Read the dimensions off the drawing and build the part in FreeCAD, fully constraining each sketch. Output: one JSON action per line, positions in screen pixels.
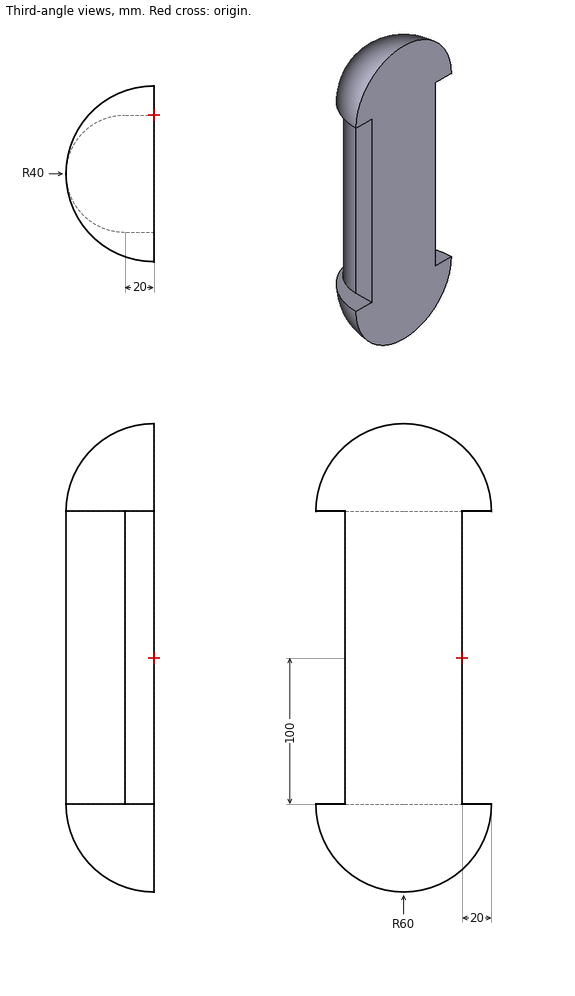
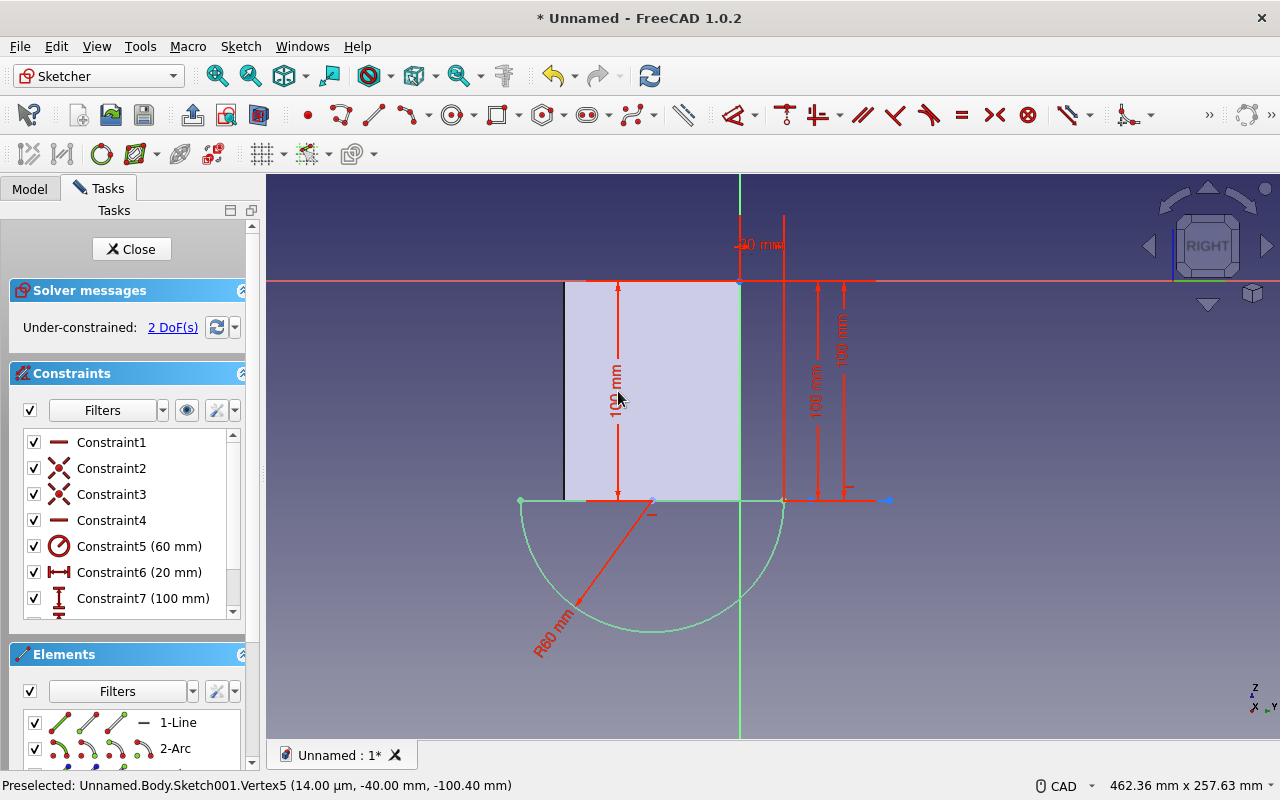
{"action": "left_click", "coordinate": [132, 249]}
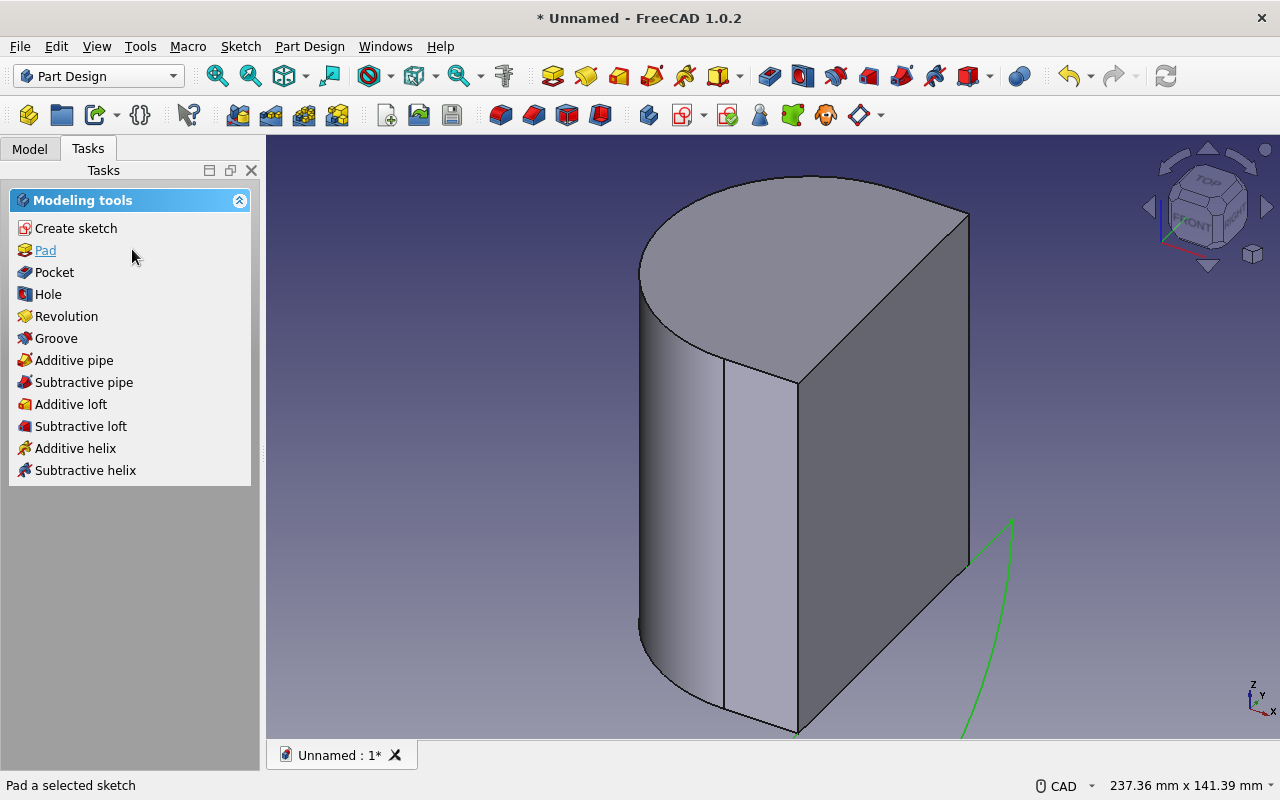
{"action": "left_click", "coordinate": [586, 76]}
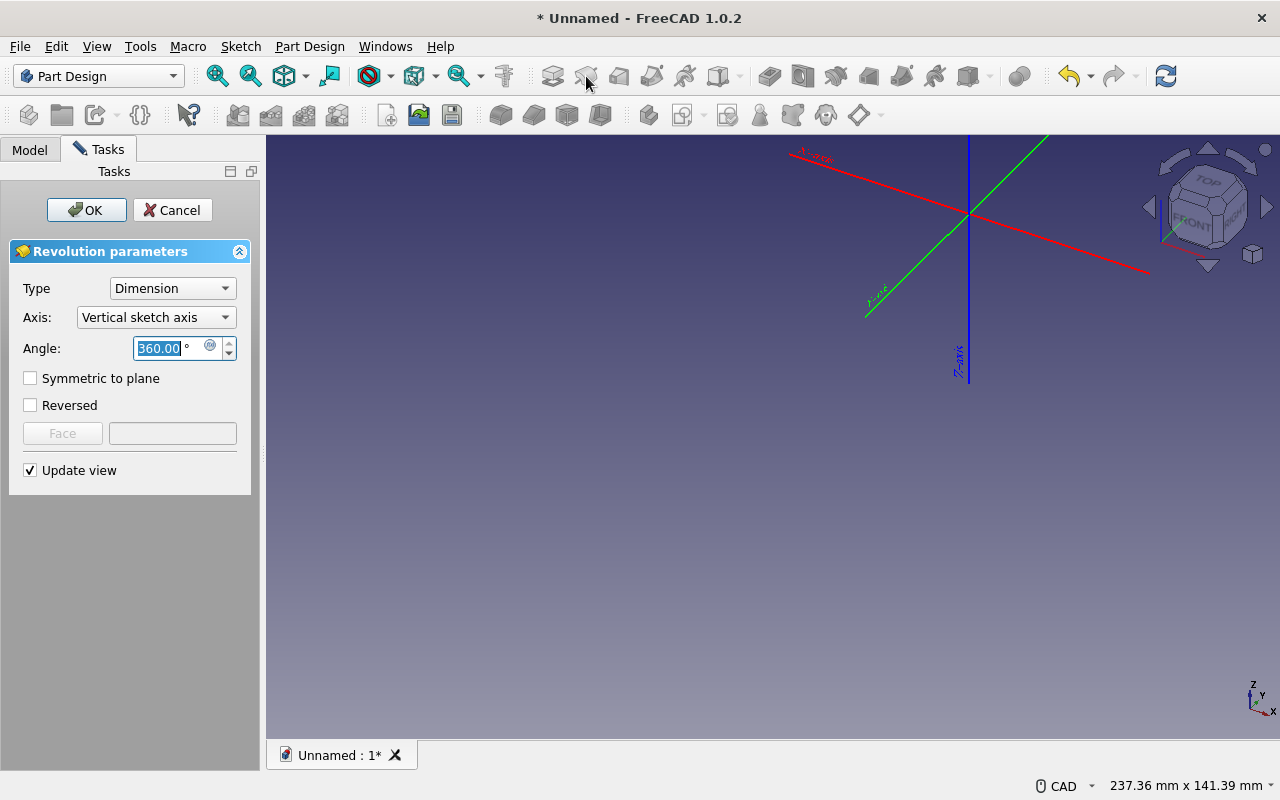
{"action": "left_click", "coordinate": [157, 318]}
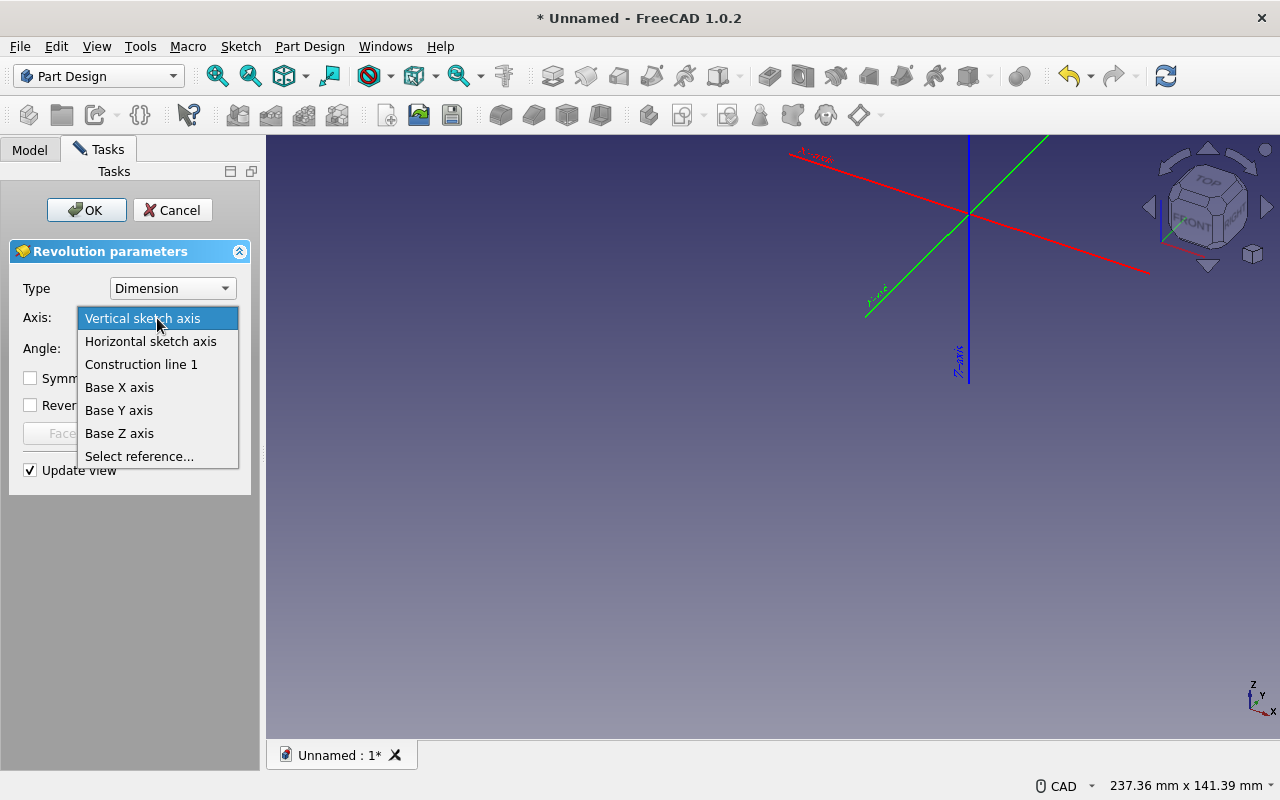
{"action": "left_click", "coordinate": [156, 364]}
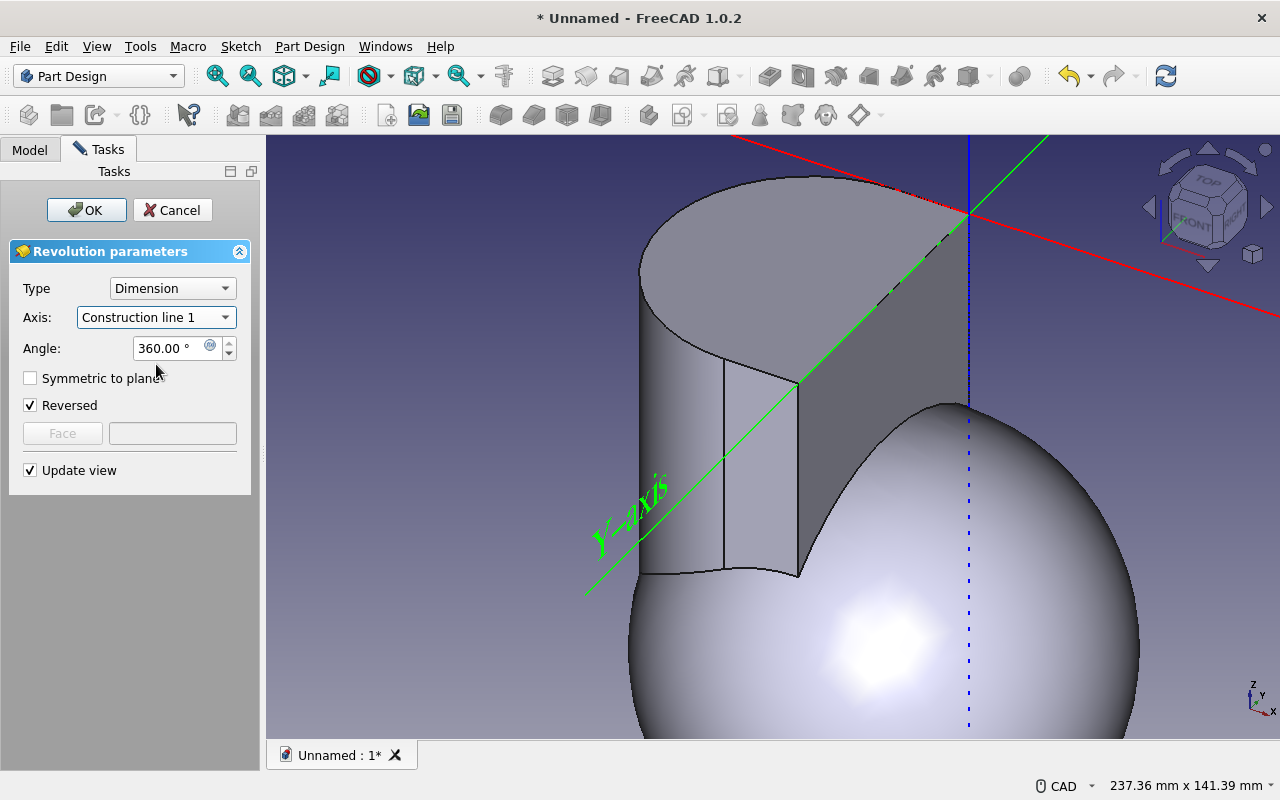
{"action": "triple_click", "coordinate": [178, 348]}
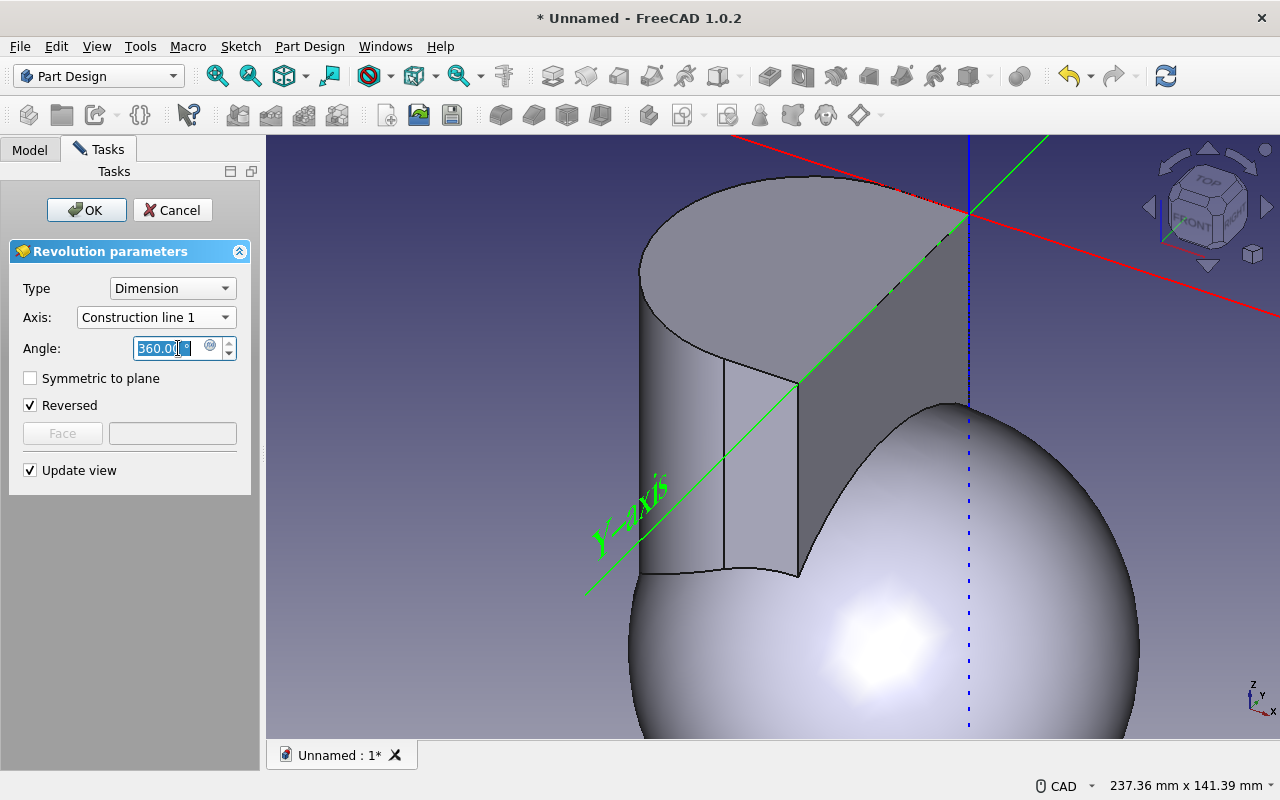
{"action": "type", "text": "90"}
{"action": "key", "text": "Tab"}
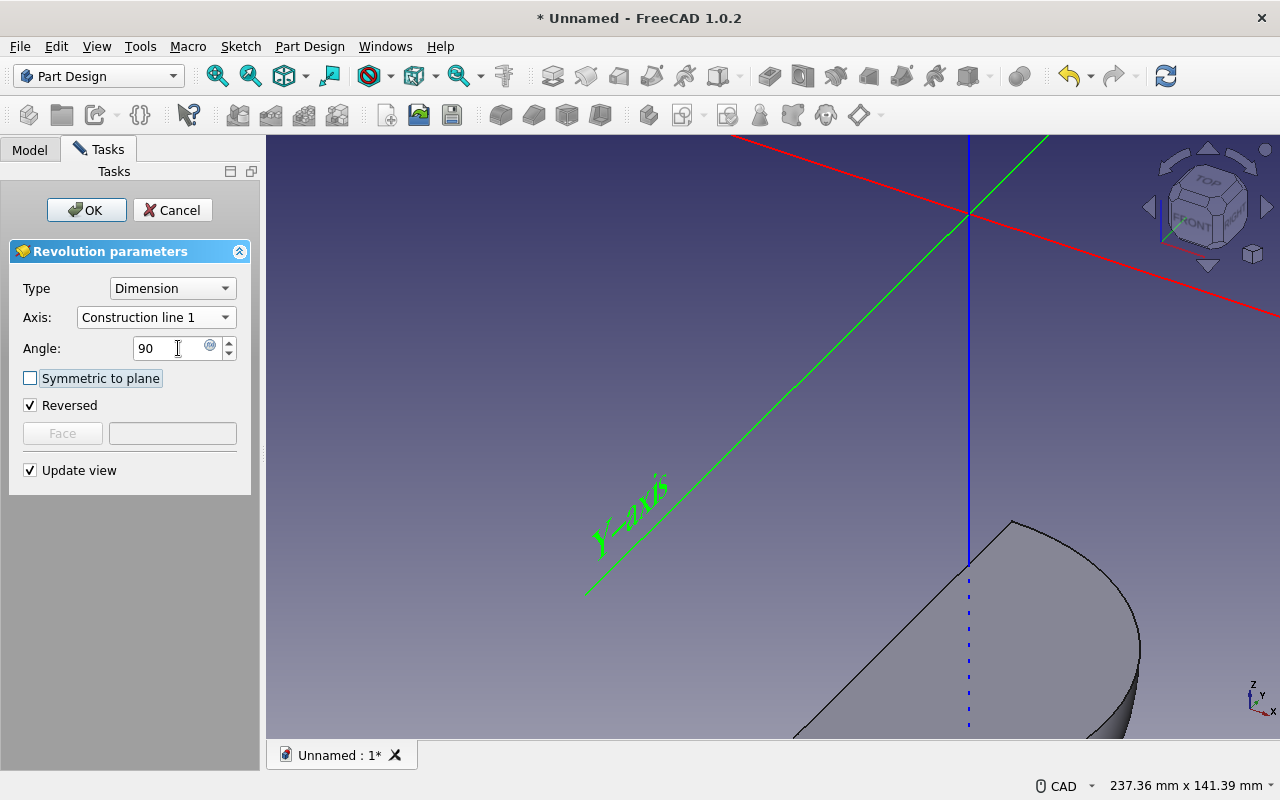
{"action": "left_click", "coordinate": [31, 405]}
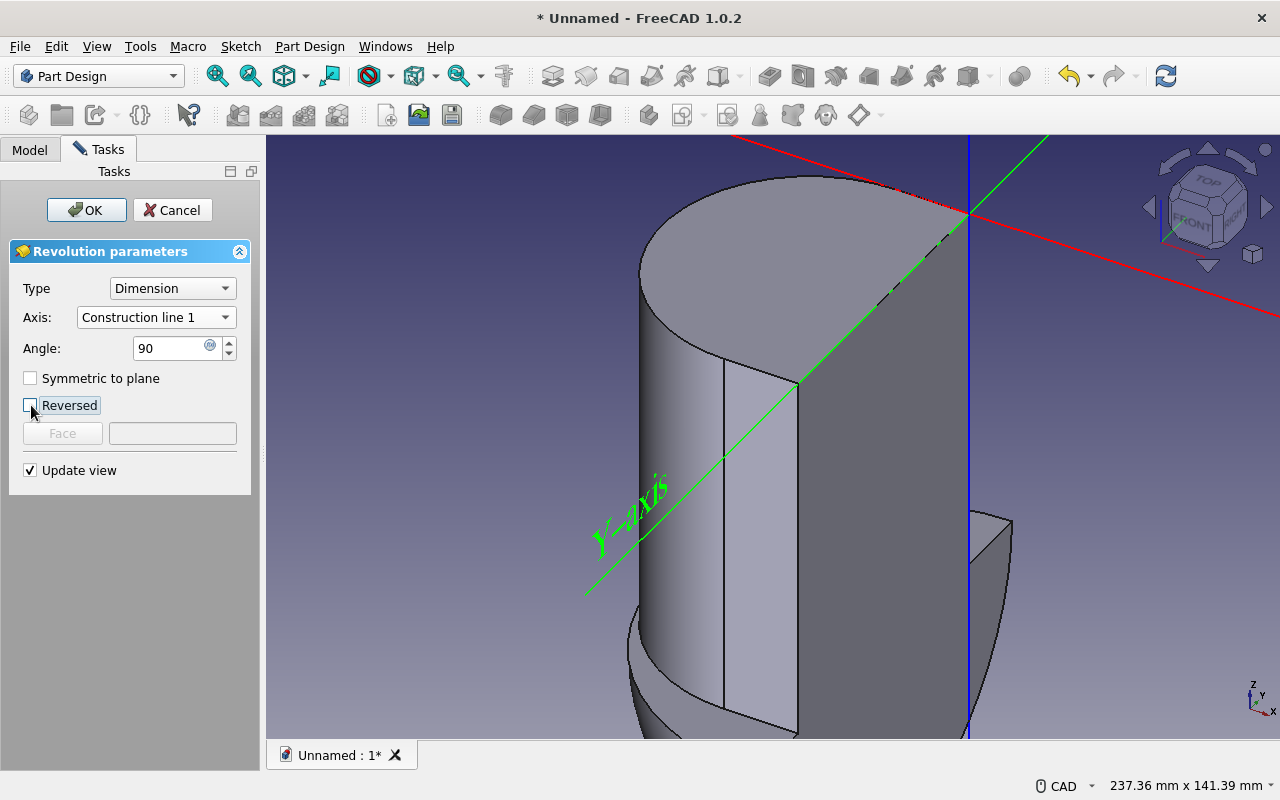
{"action": "left_click", "coordinate": [87, 210]}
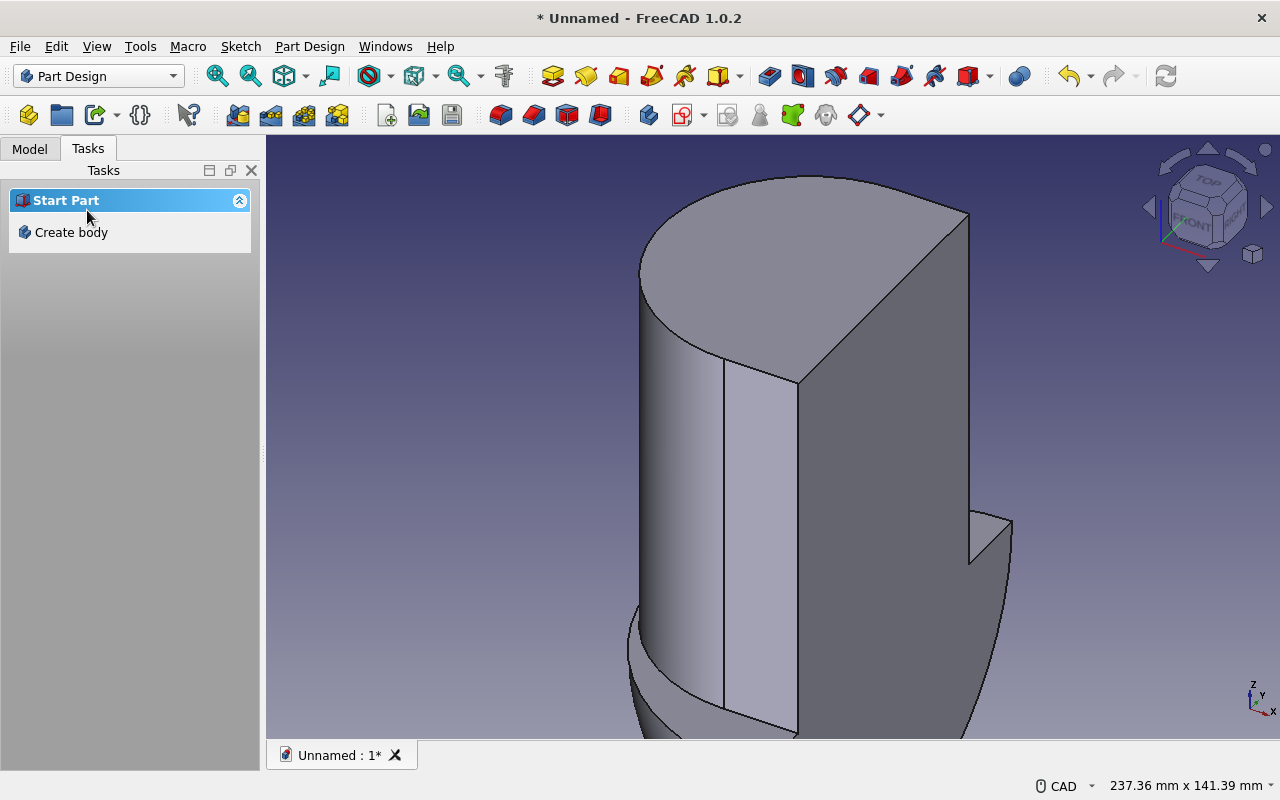
{"action": "key", "text": "v f"}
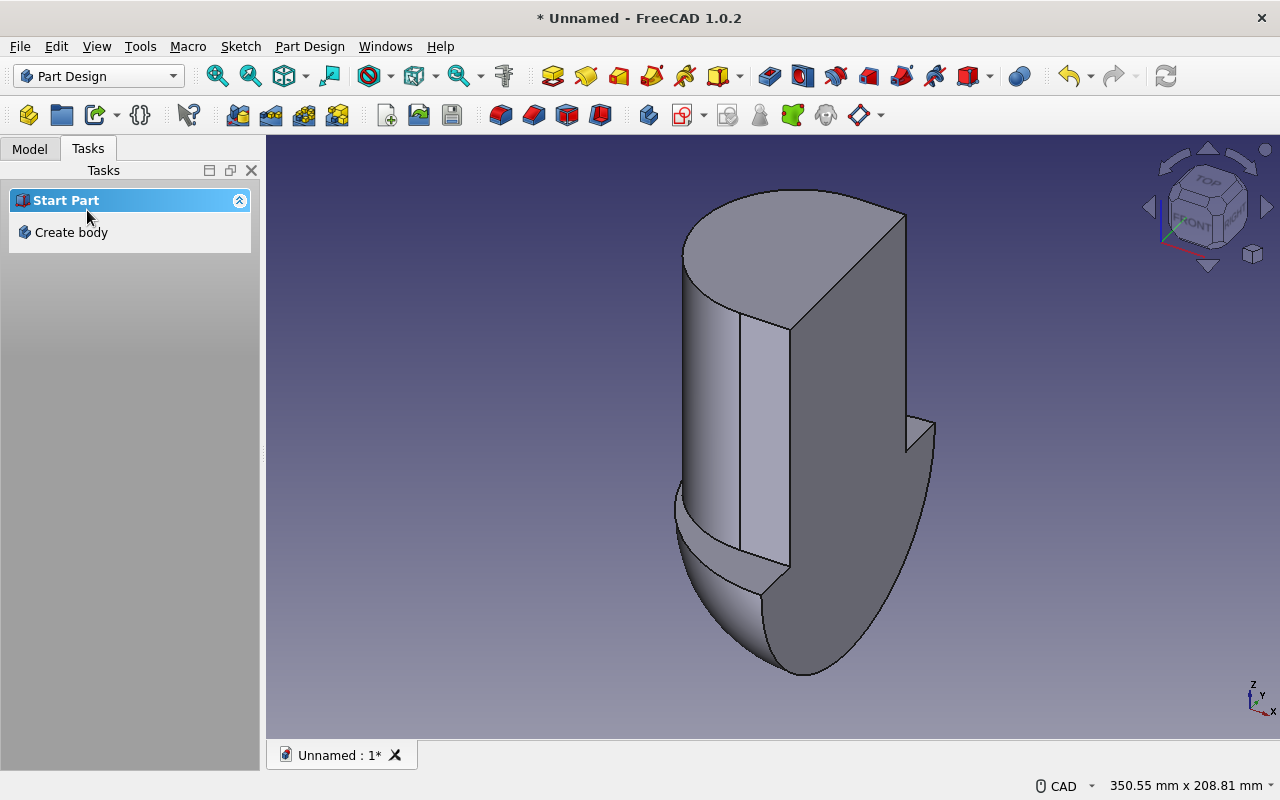
{"action": "left_click", "coordinate": [30, 148]}